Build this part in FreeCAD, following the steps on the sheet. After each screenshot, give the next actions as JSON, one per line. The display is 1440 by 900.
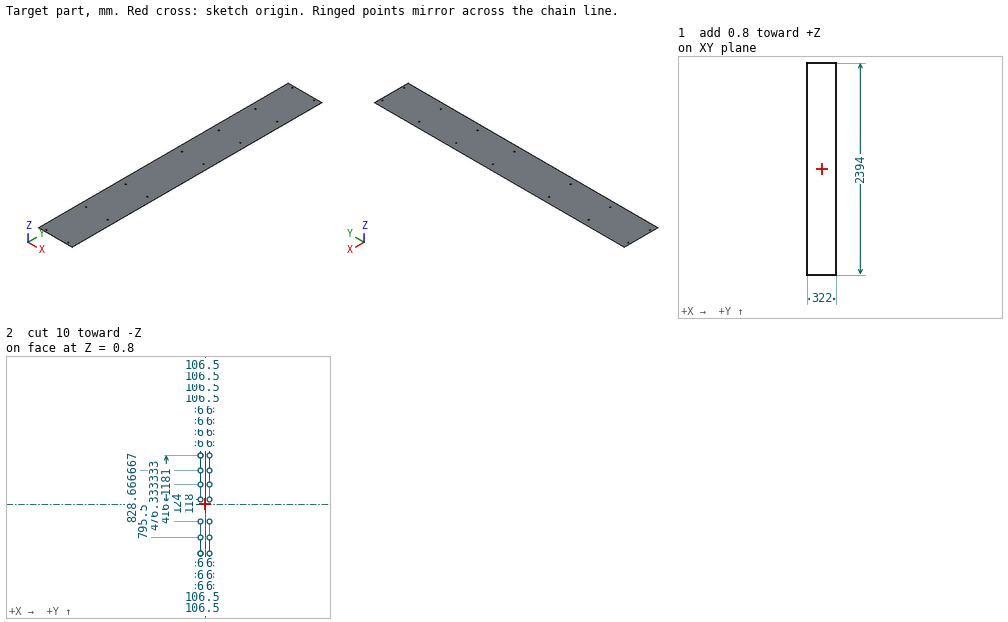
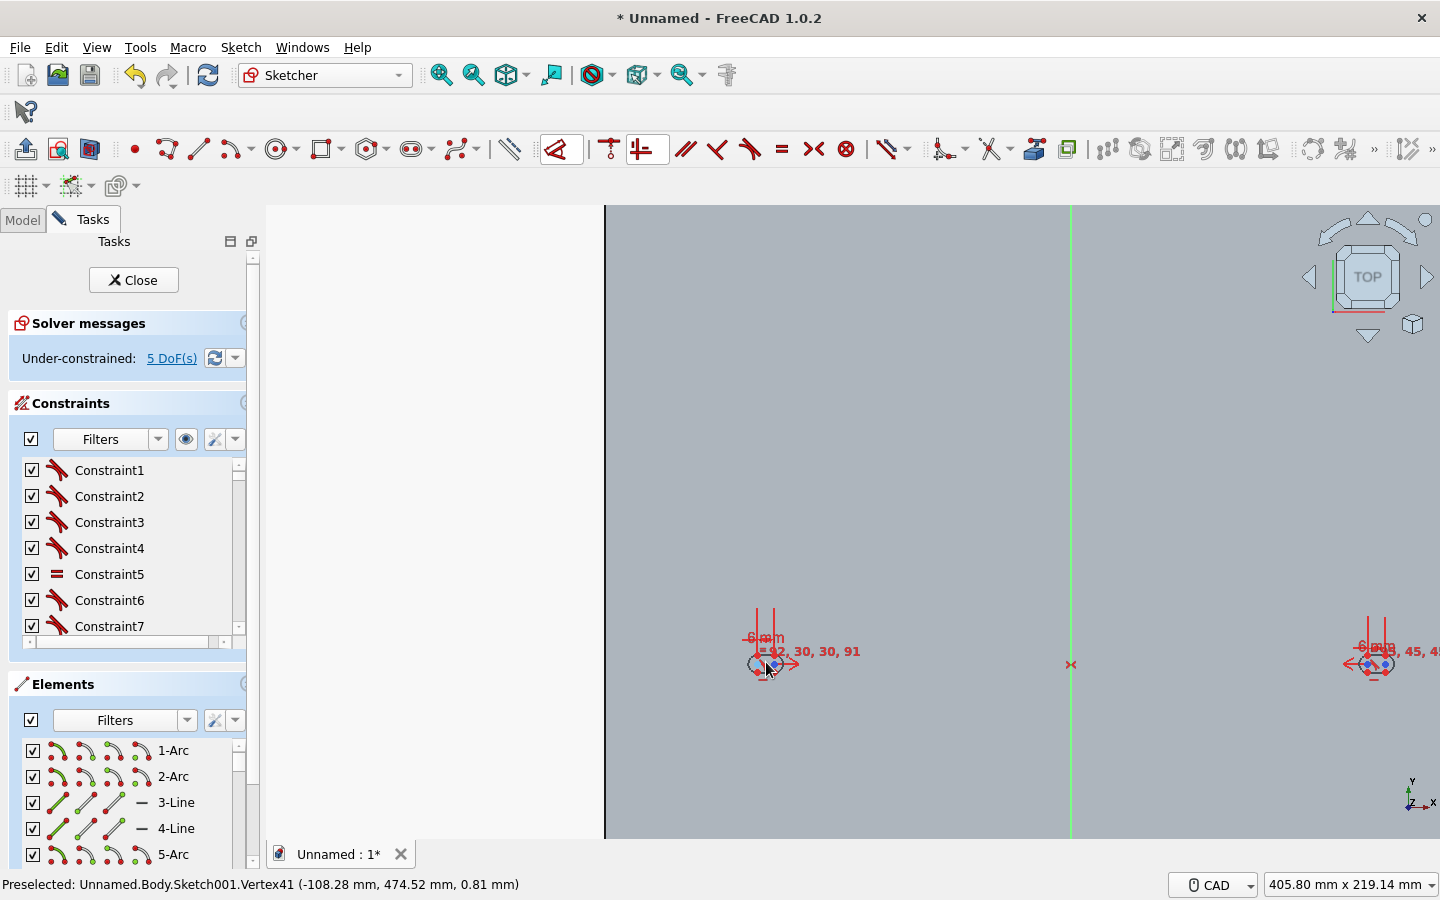
{"action": "left_click", "coordinate": [757, 655]}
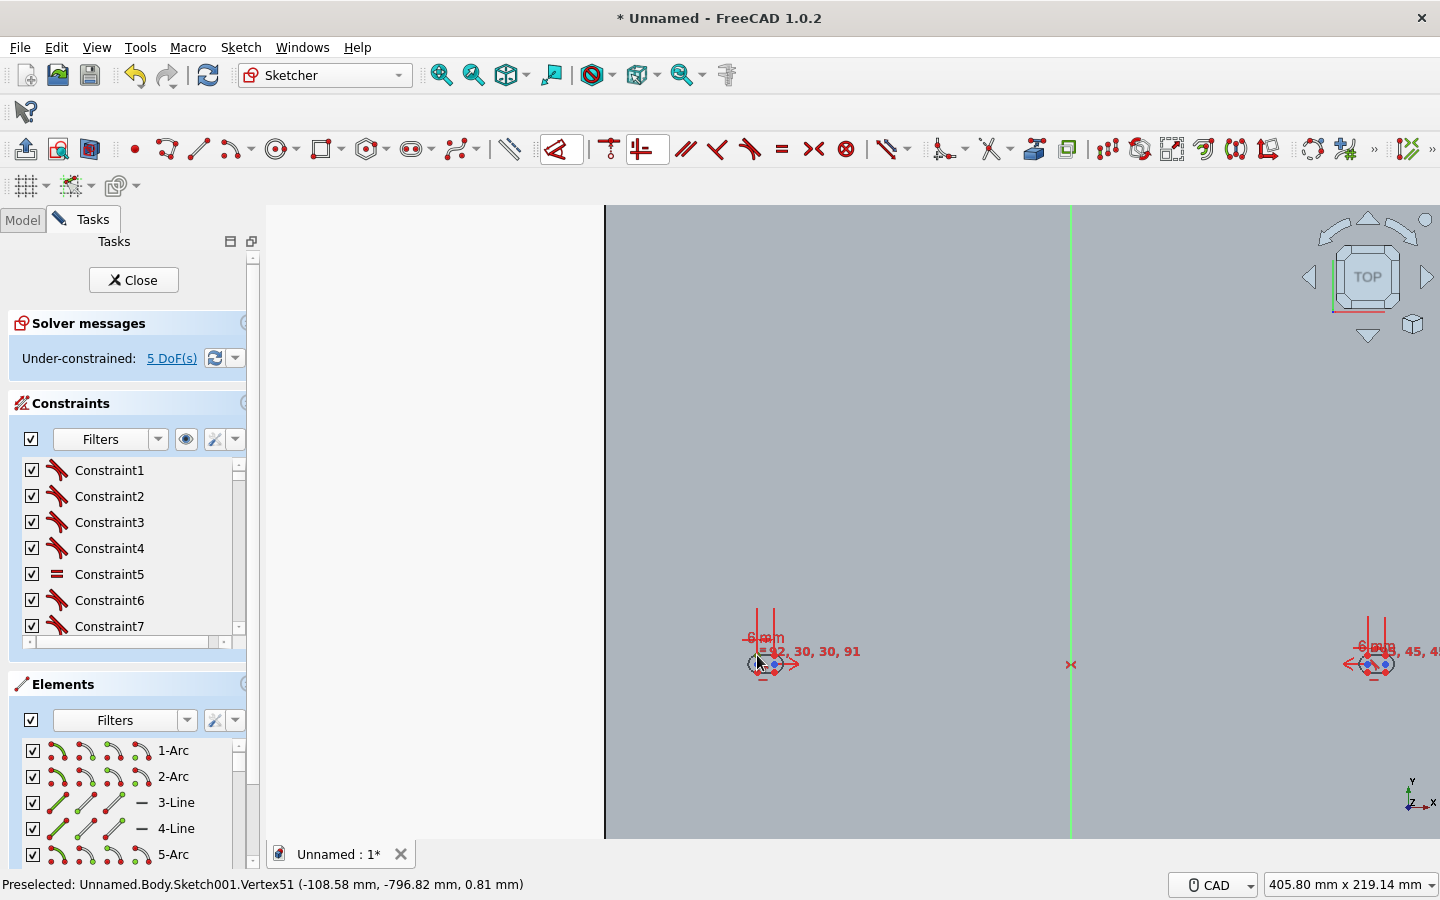
{"action": "key", "text": "l"}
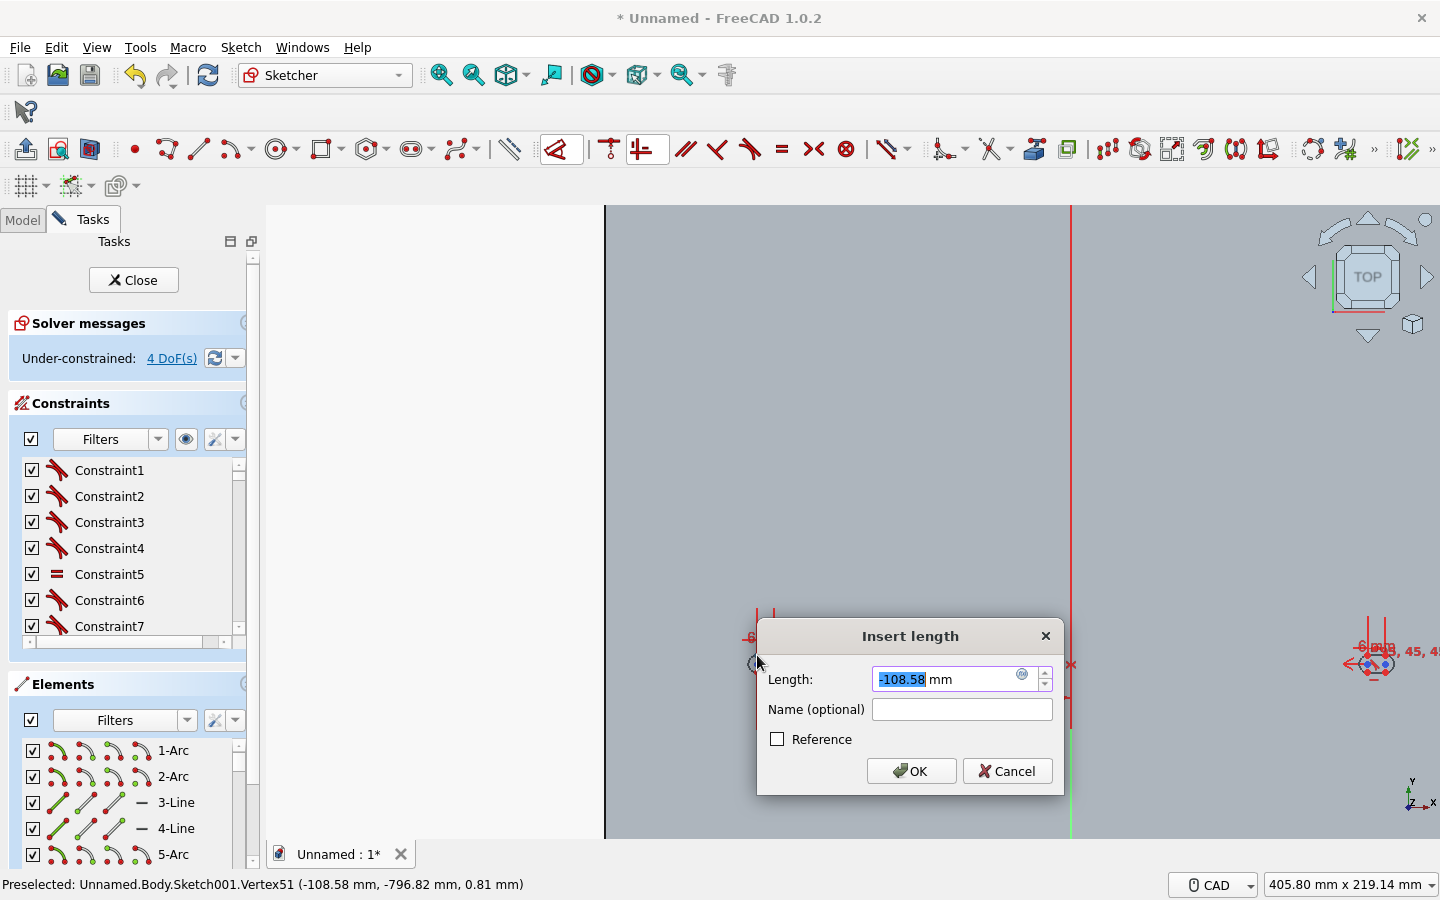
{"action": "type", "text": "-106.5"}
{"action": "key", "text": "Return"}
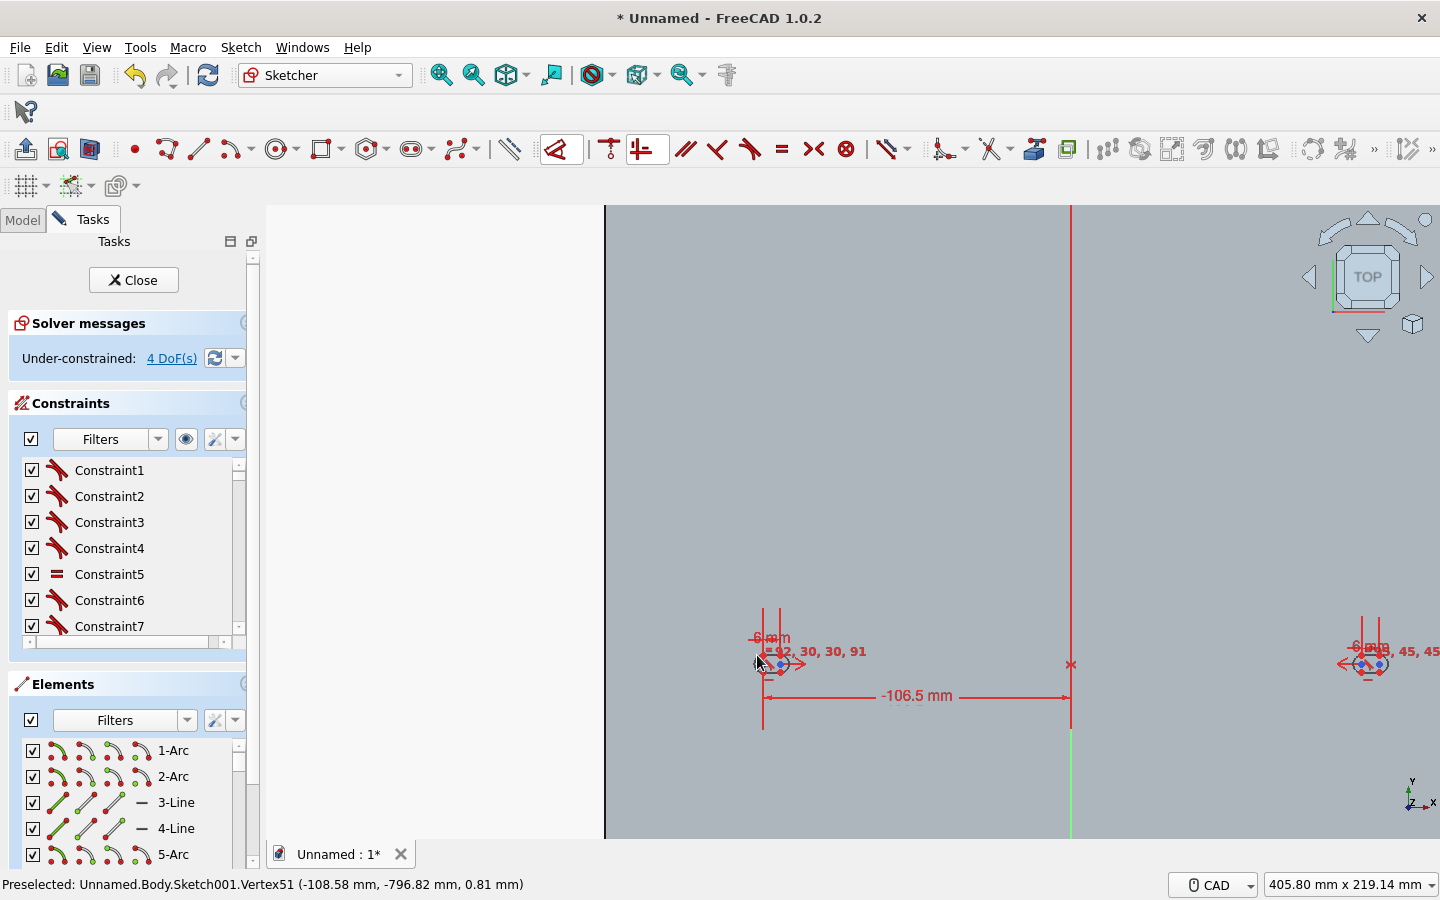
{"action": "left_click", "coordinate": [763, 655]}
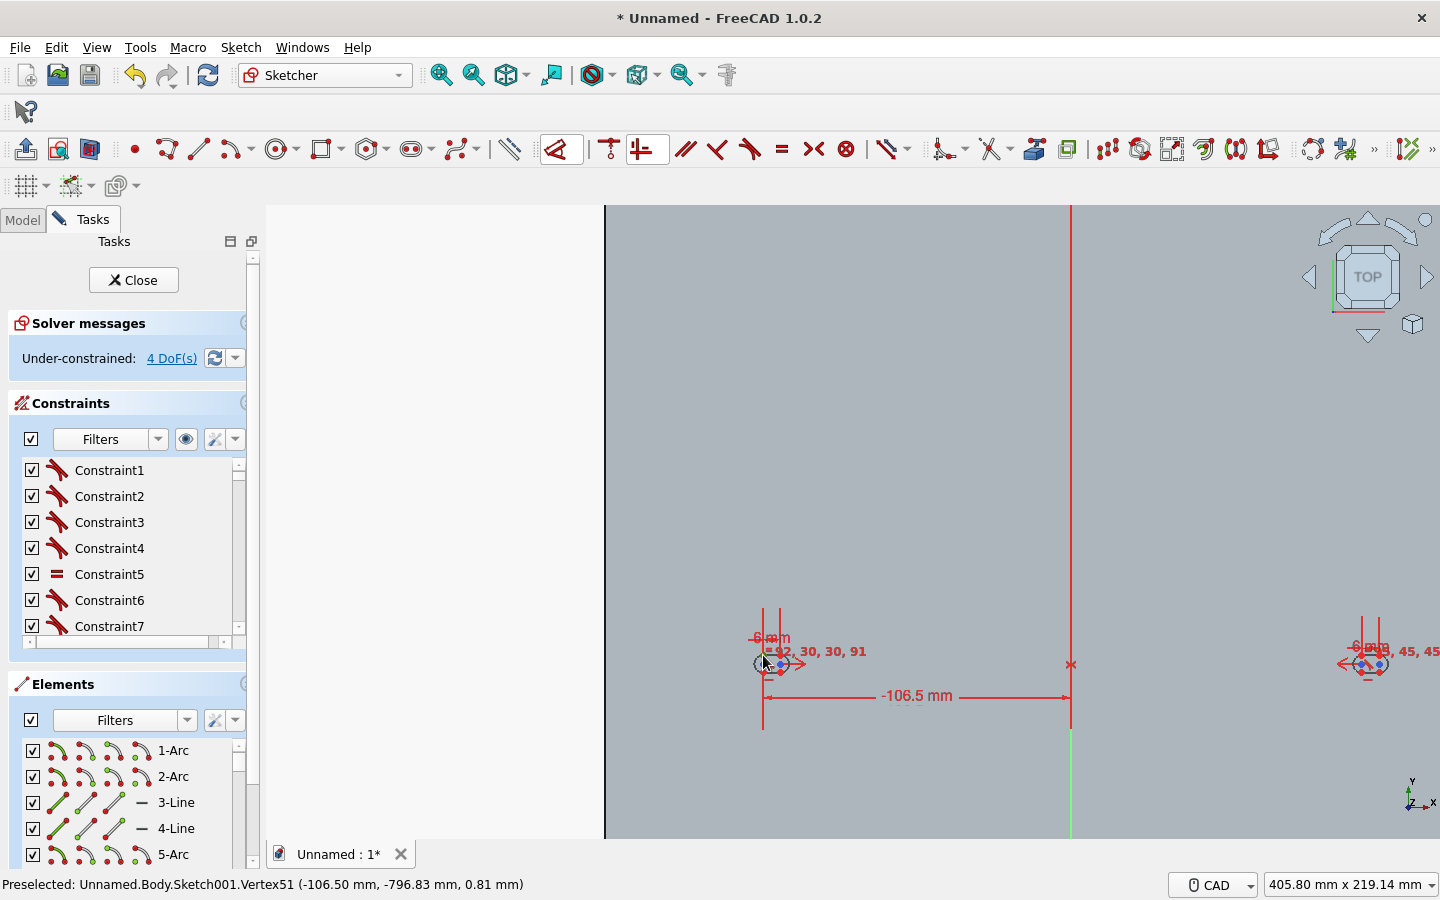
{"action": "key", "text": "i"}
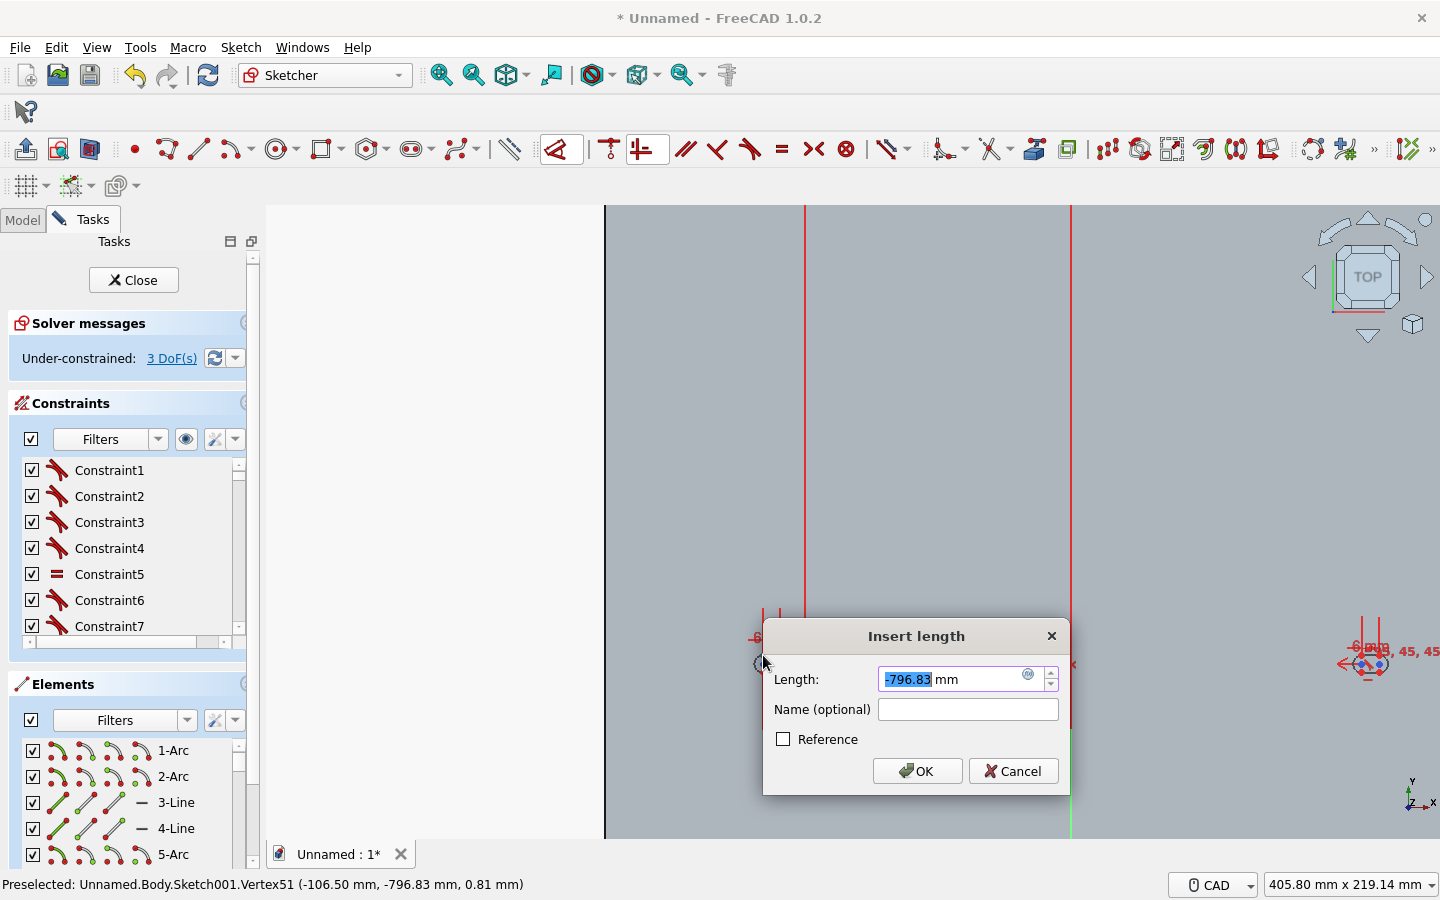
{"action": "type", "text": "-795.5"}
{"action": "key", "text": "Return"}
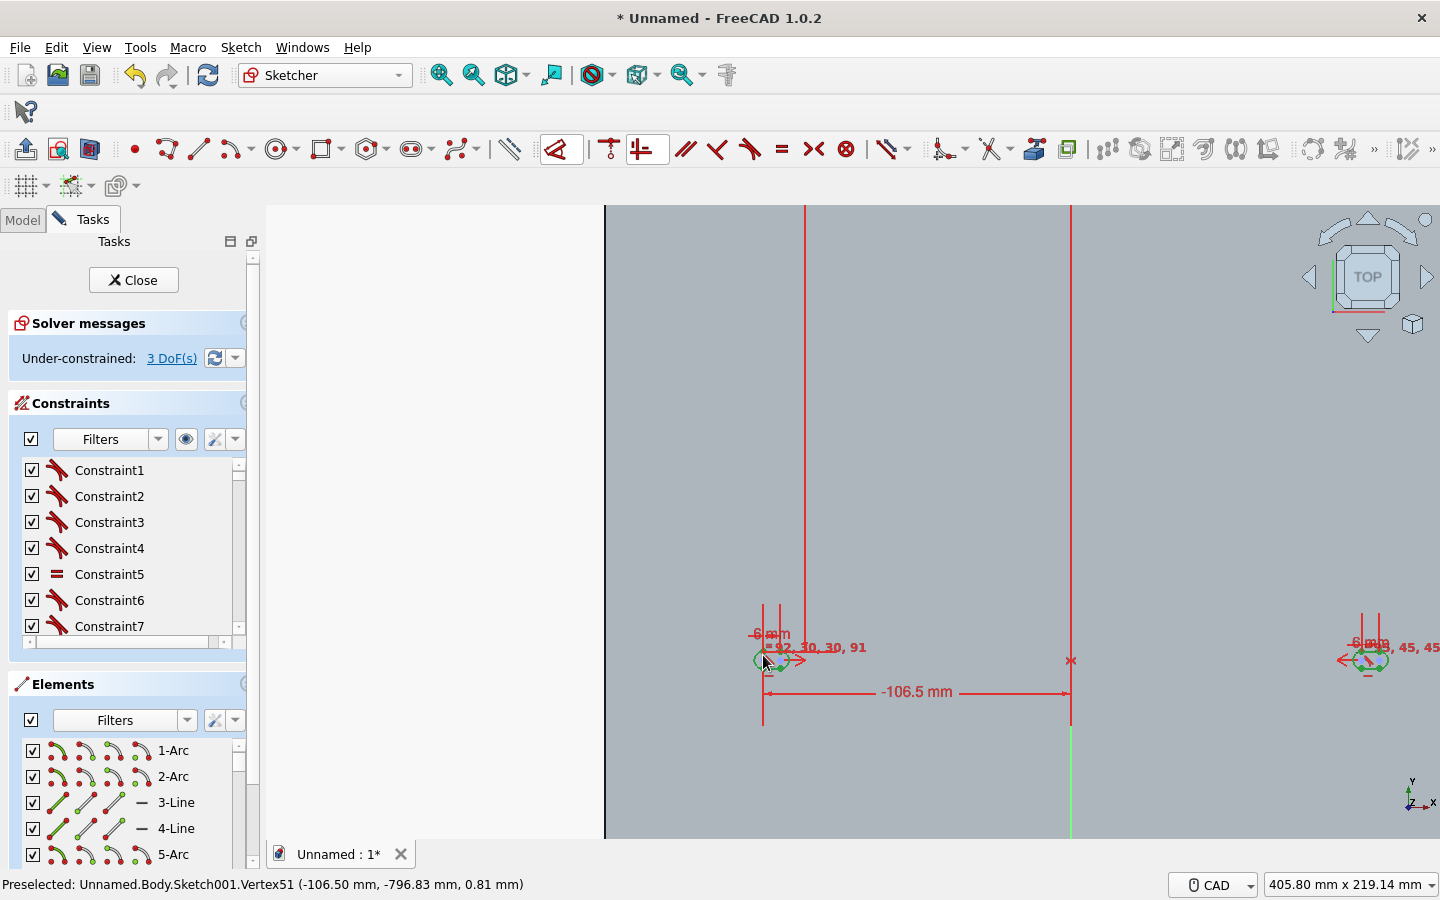
{"action": "scroll", "coordinate": [766, 663], "scroll_direction": "down", "scroll_amount": 14}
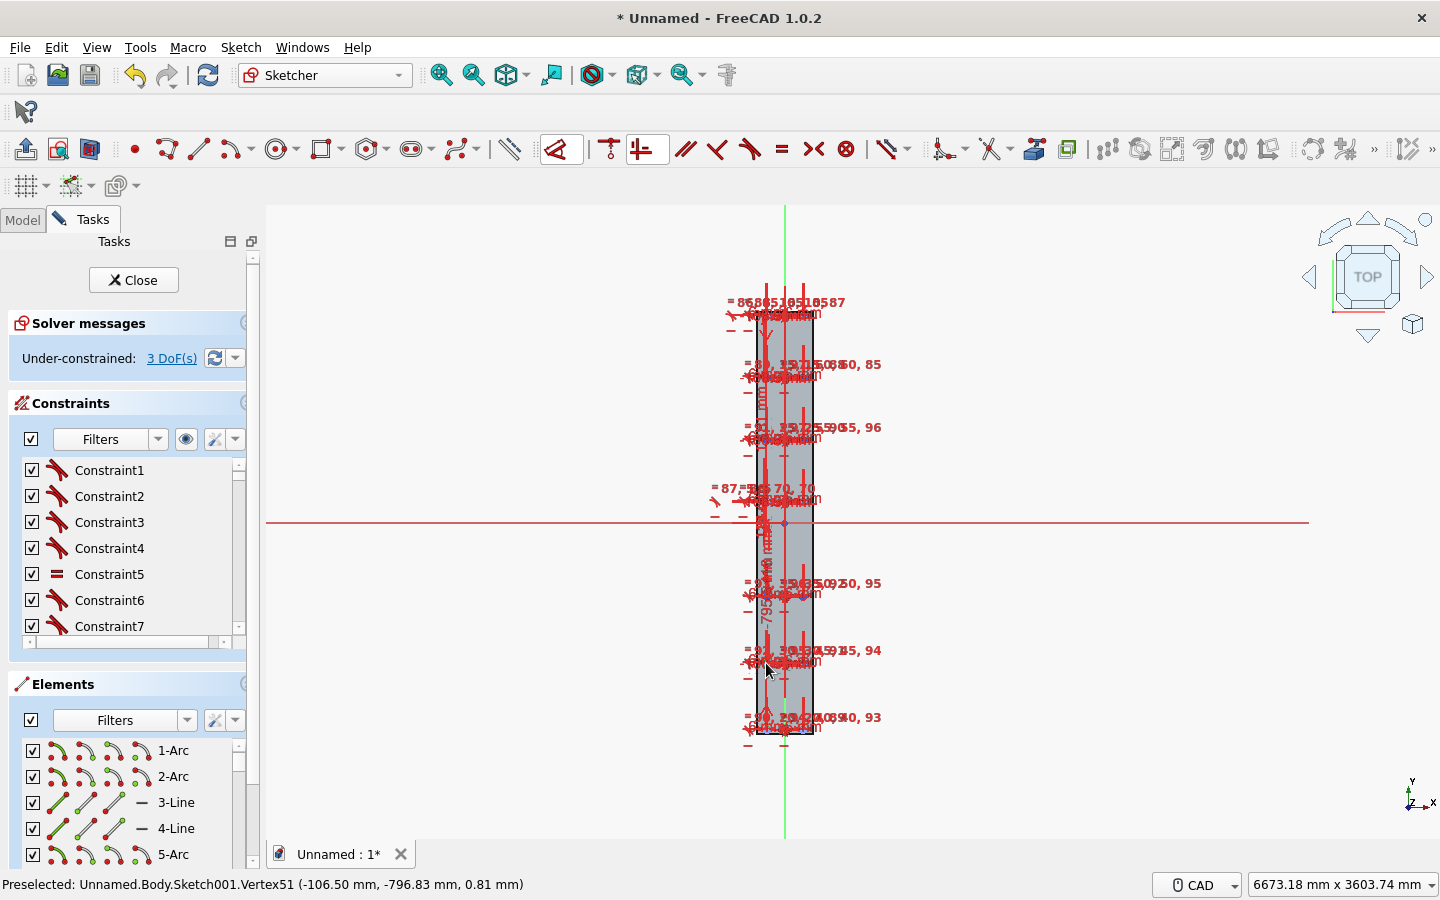
{"action": "scroll", "coordinate": [766, 596], "scroll_direction": "up", "scroll_amount": 14}